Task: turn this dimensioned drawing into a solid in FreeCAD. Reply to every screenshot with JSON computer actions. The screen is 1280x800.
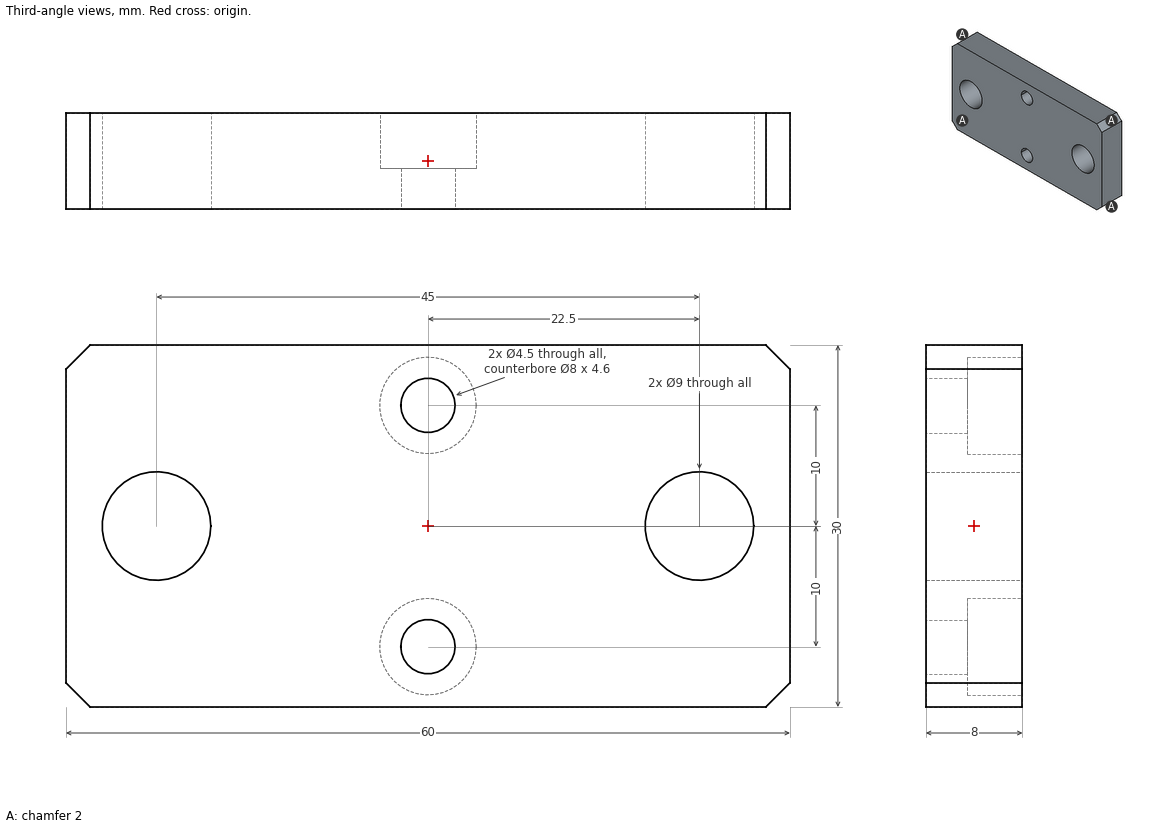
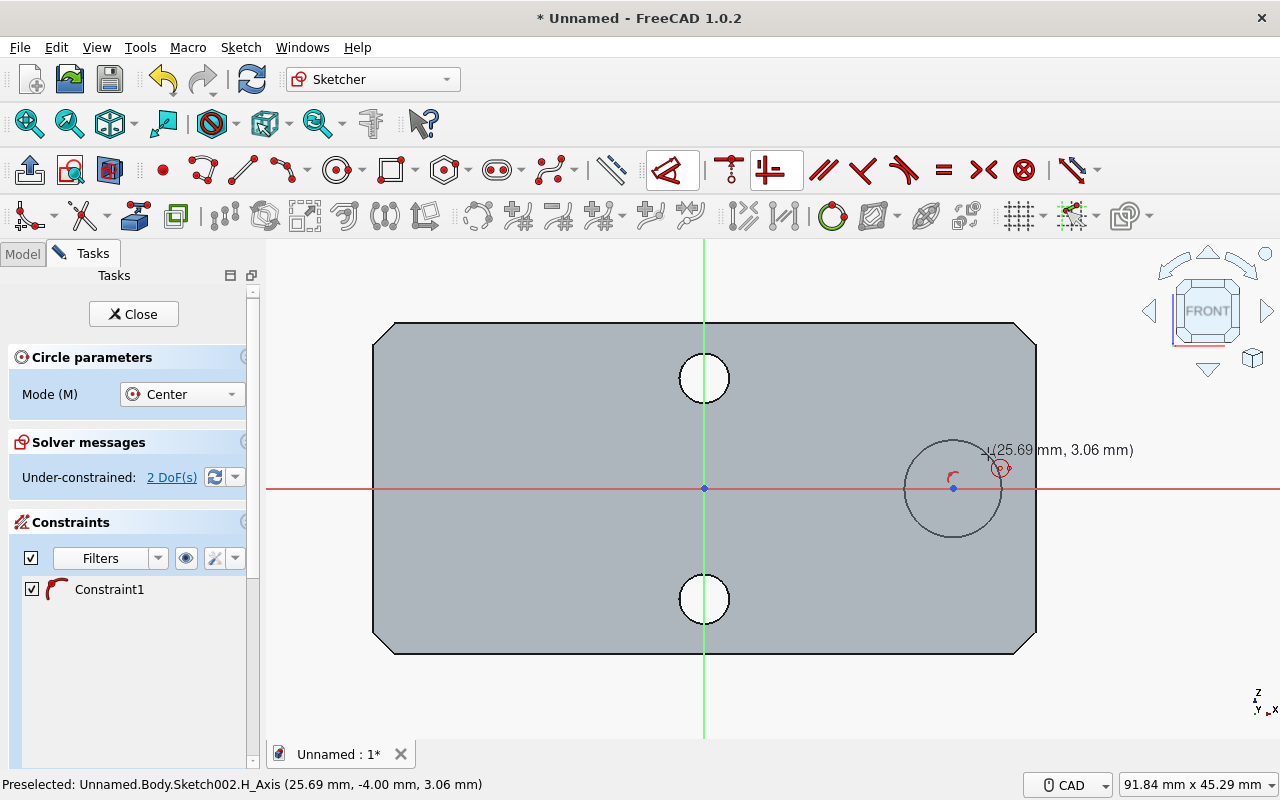
{"action": "left_click", "coordinate": [456, 489]}
{"action": "left_click", "coordinate": [491, 454]}
{"action": "key", "text": "Escape"}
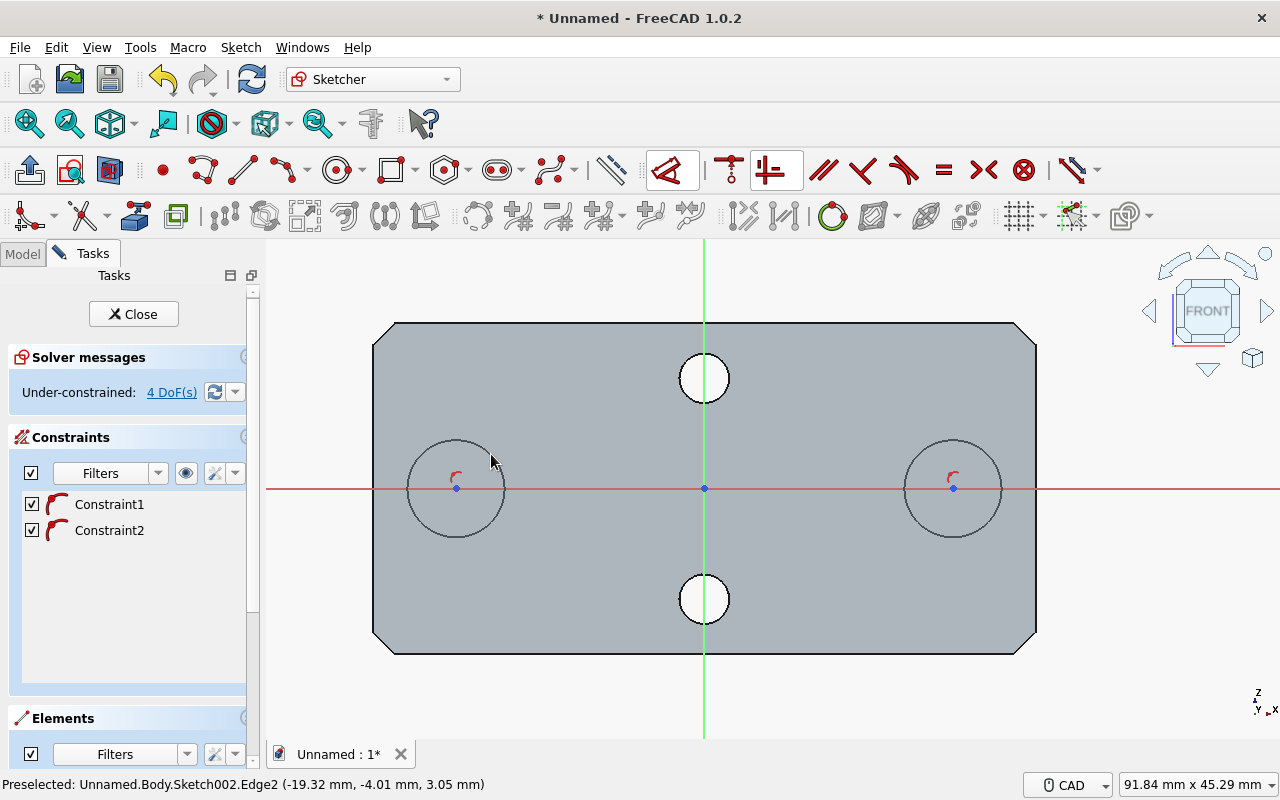
{"action": "left_click", "coordinate": [987, 454]}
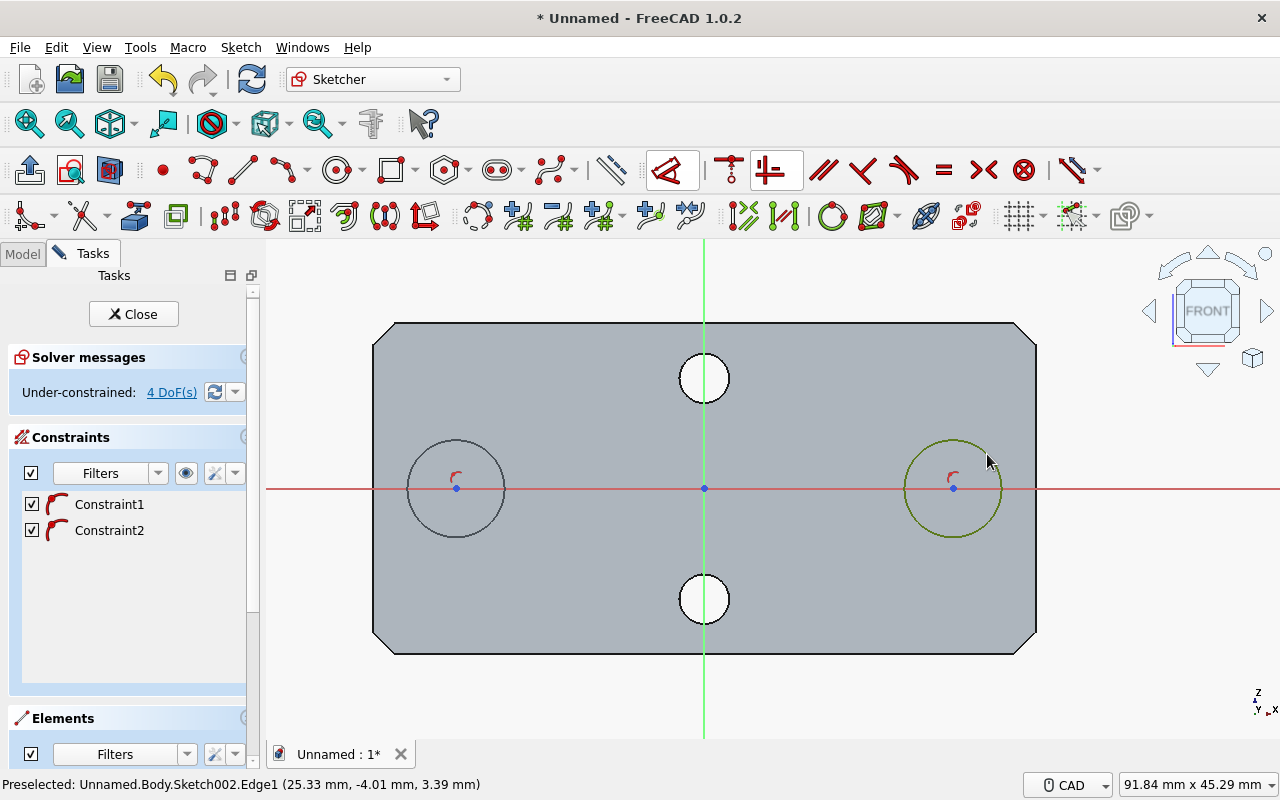
{"action": "left_click", "coordinate": [490, 454]}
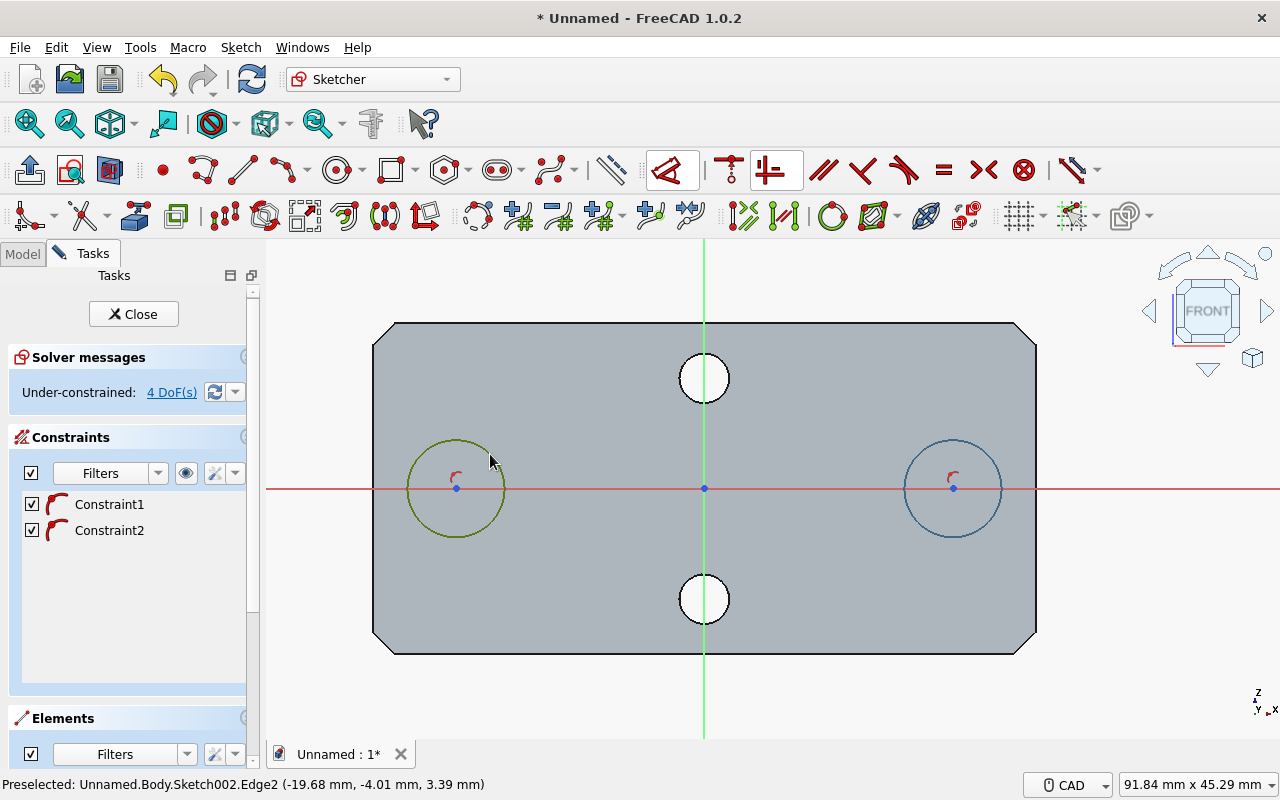
{"action": "left_click", "coordinate": [944, 170]}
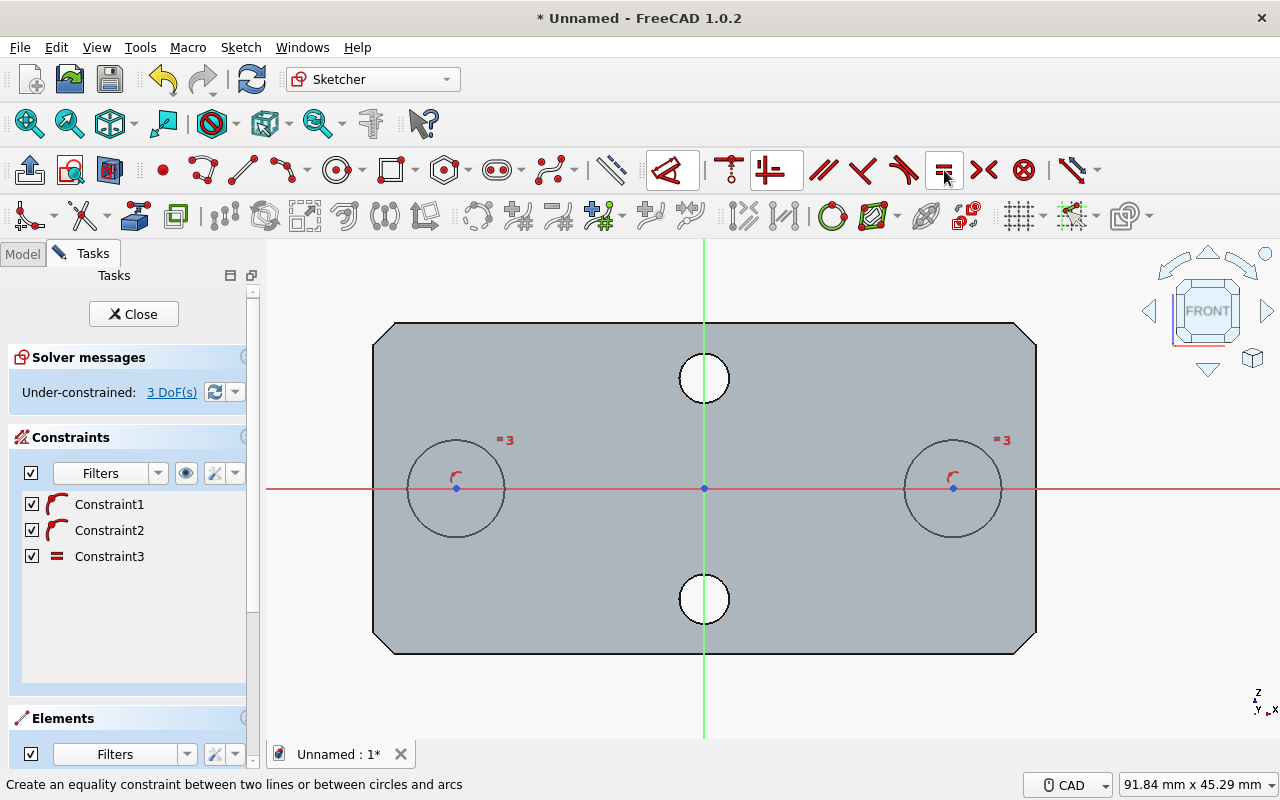
{"action": "left_click", "coordinate": [987, 454]}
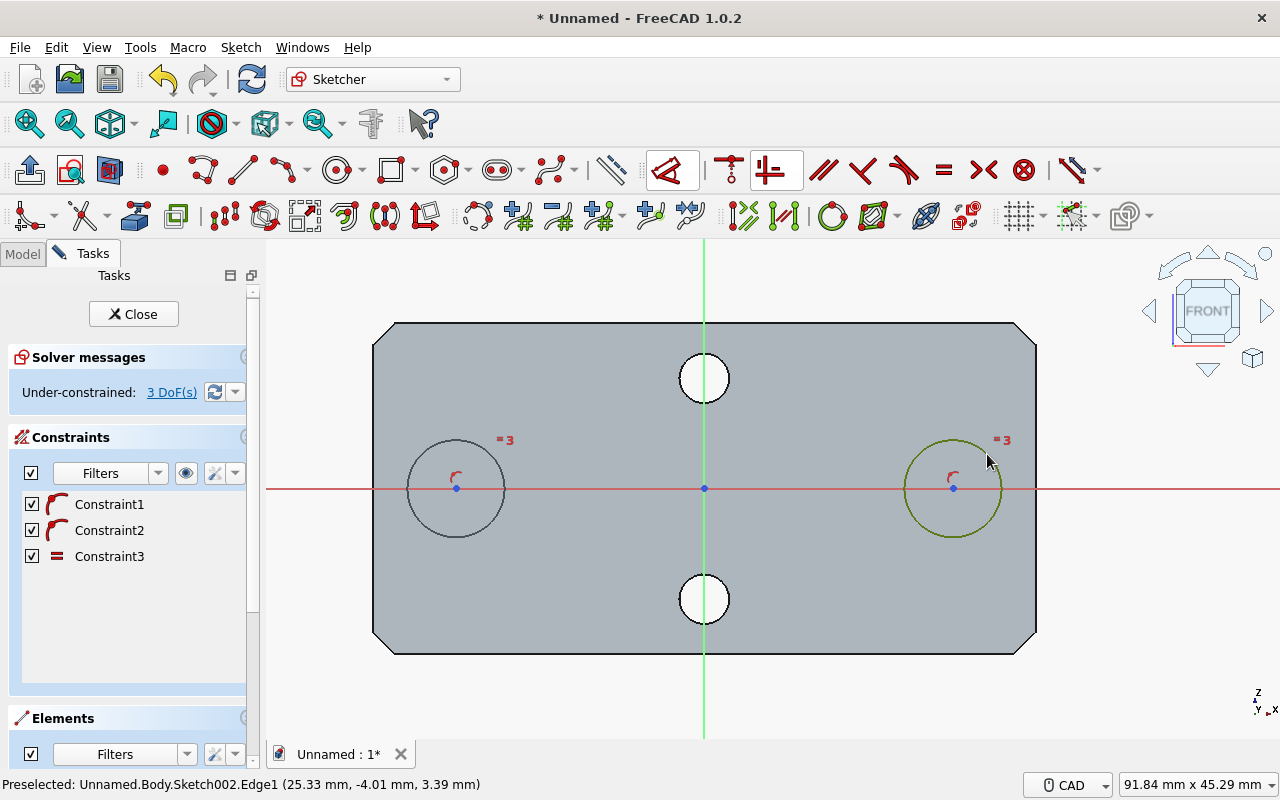
{"action": "key", "text": "k o"}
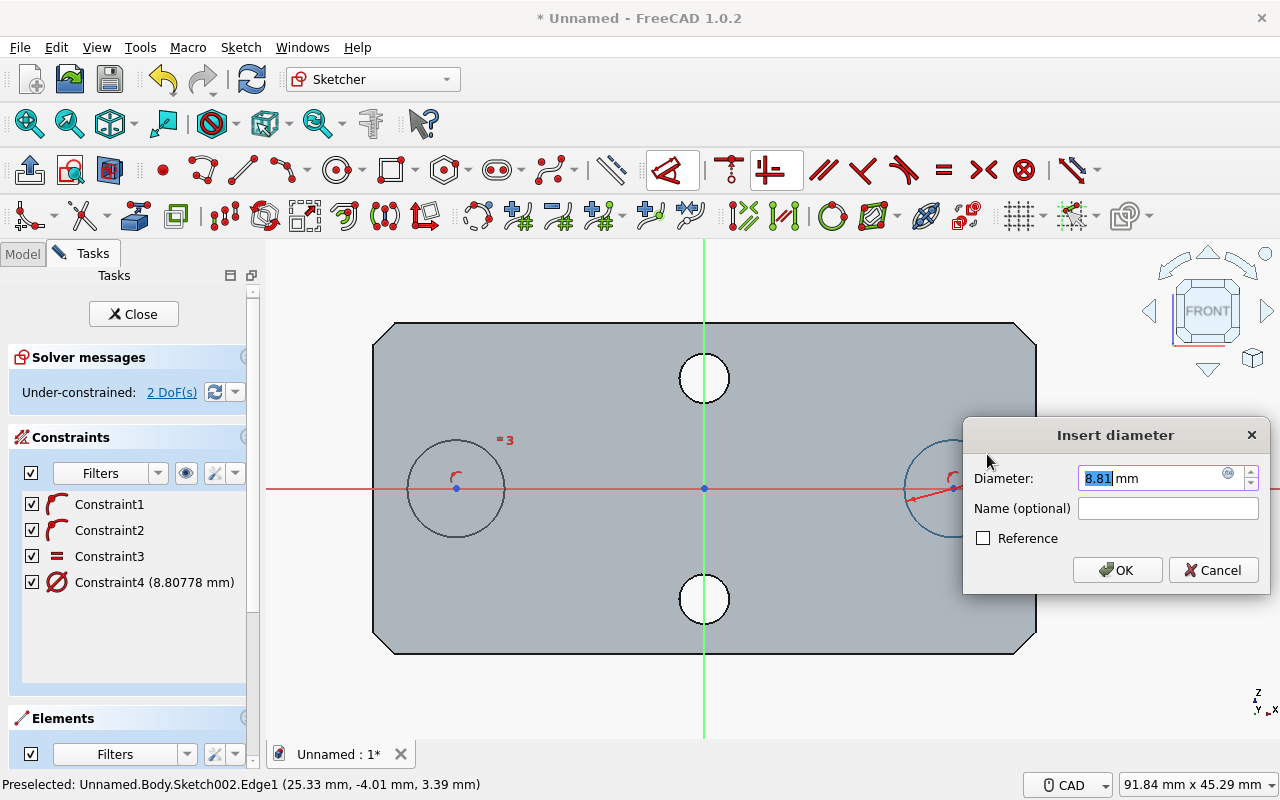
{"action": "type", "text": "9"}
{"action": "key", "text": "Return"}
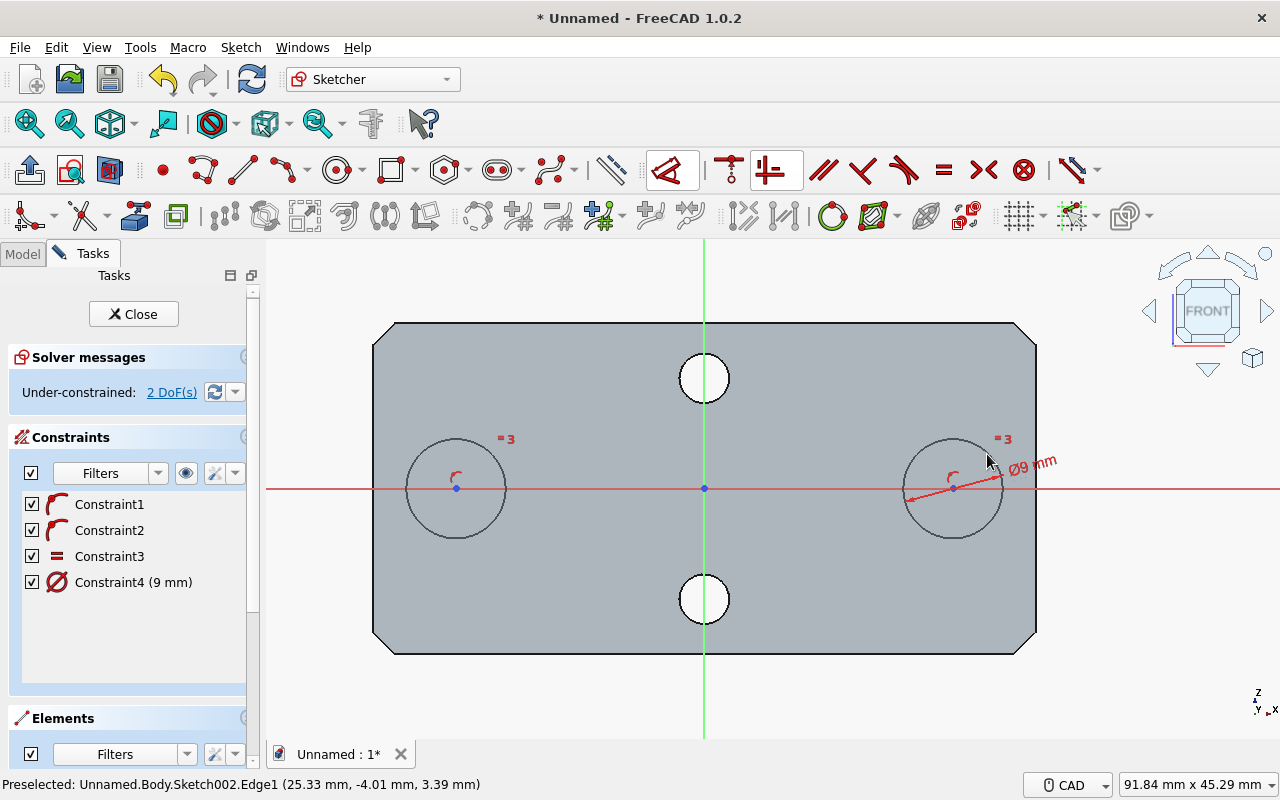
{"action": "left_click", "coordinate": [953, 489]}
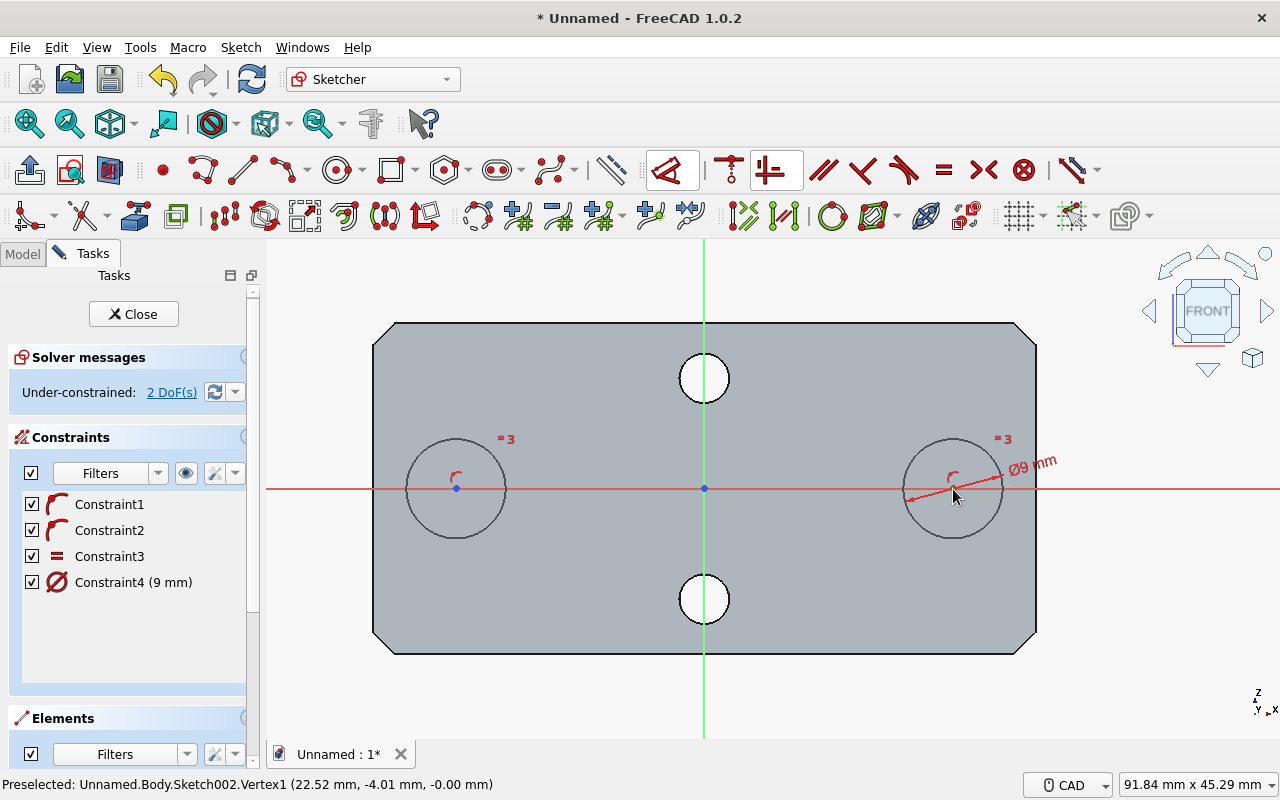
{"action": "left_click", "coordinate": [456, 489]}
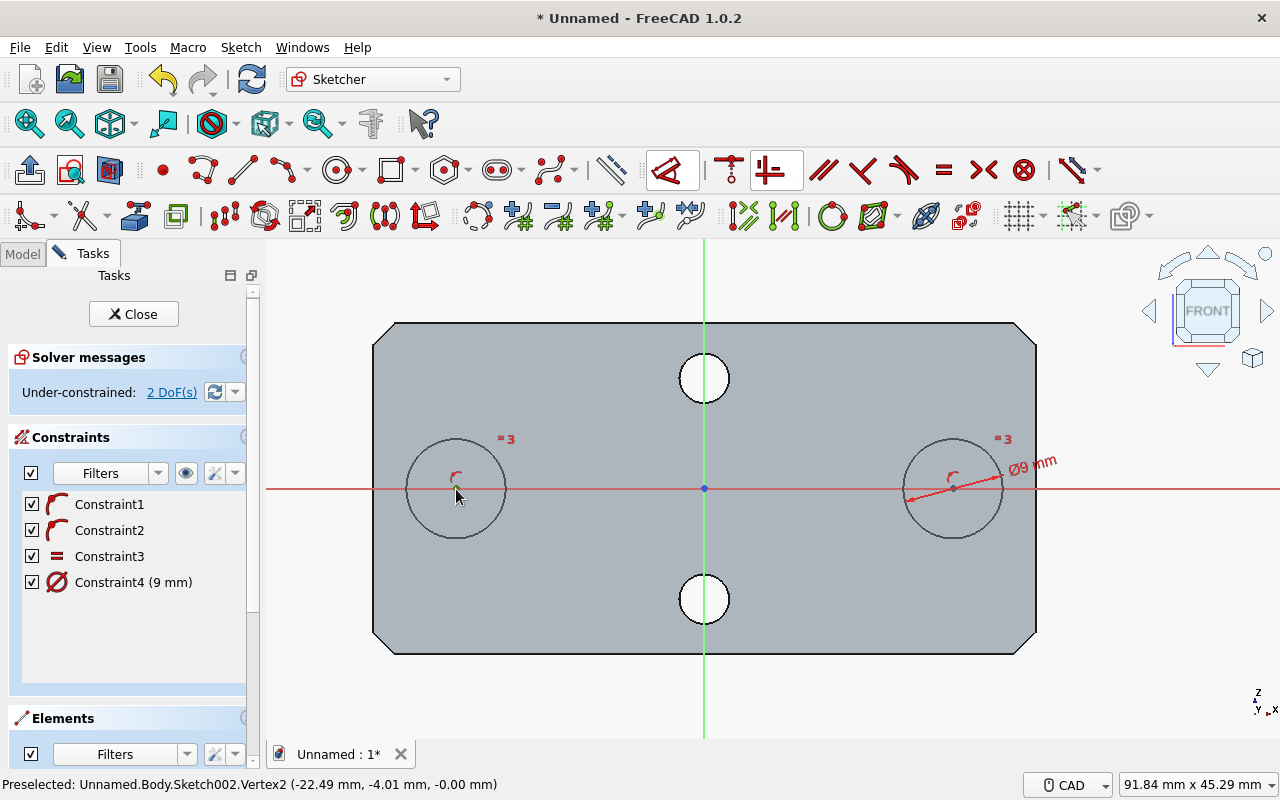
{"action": "key", "text": "l"}